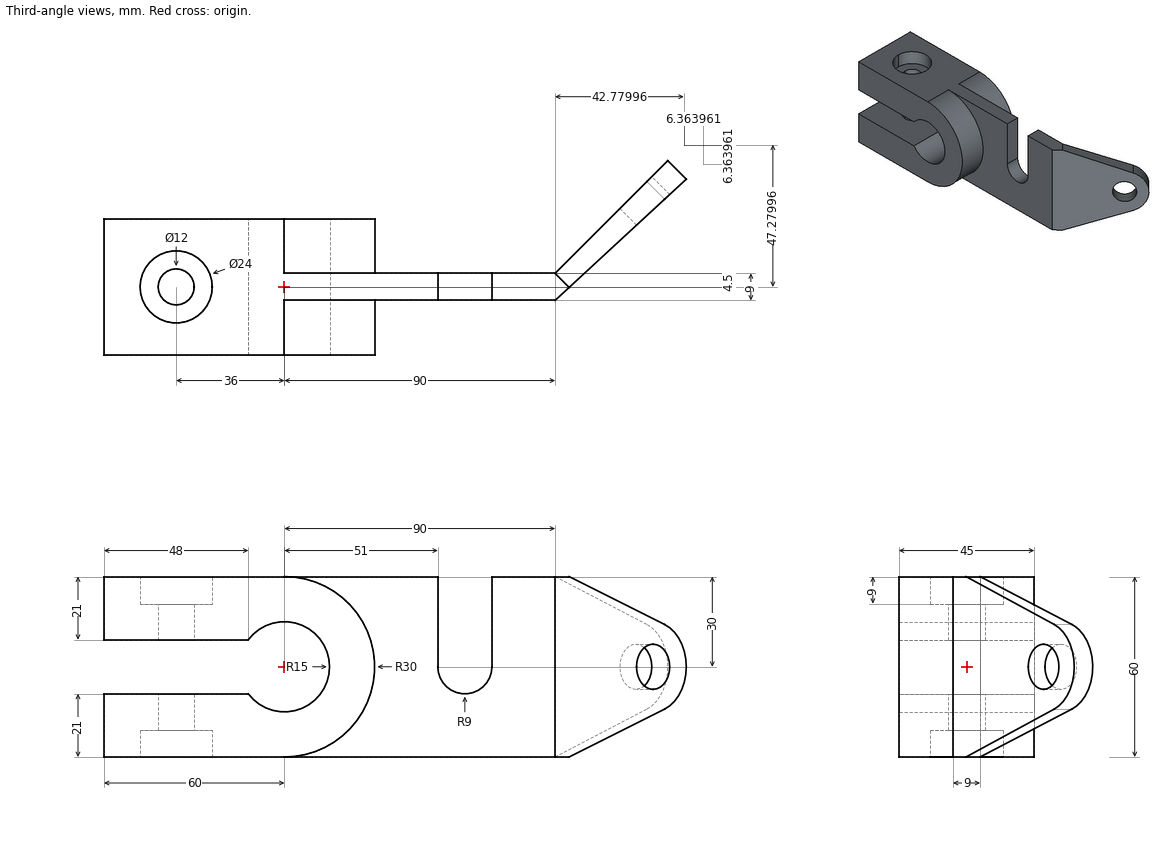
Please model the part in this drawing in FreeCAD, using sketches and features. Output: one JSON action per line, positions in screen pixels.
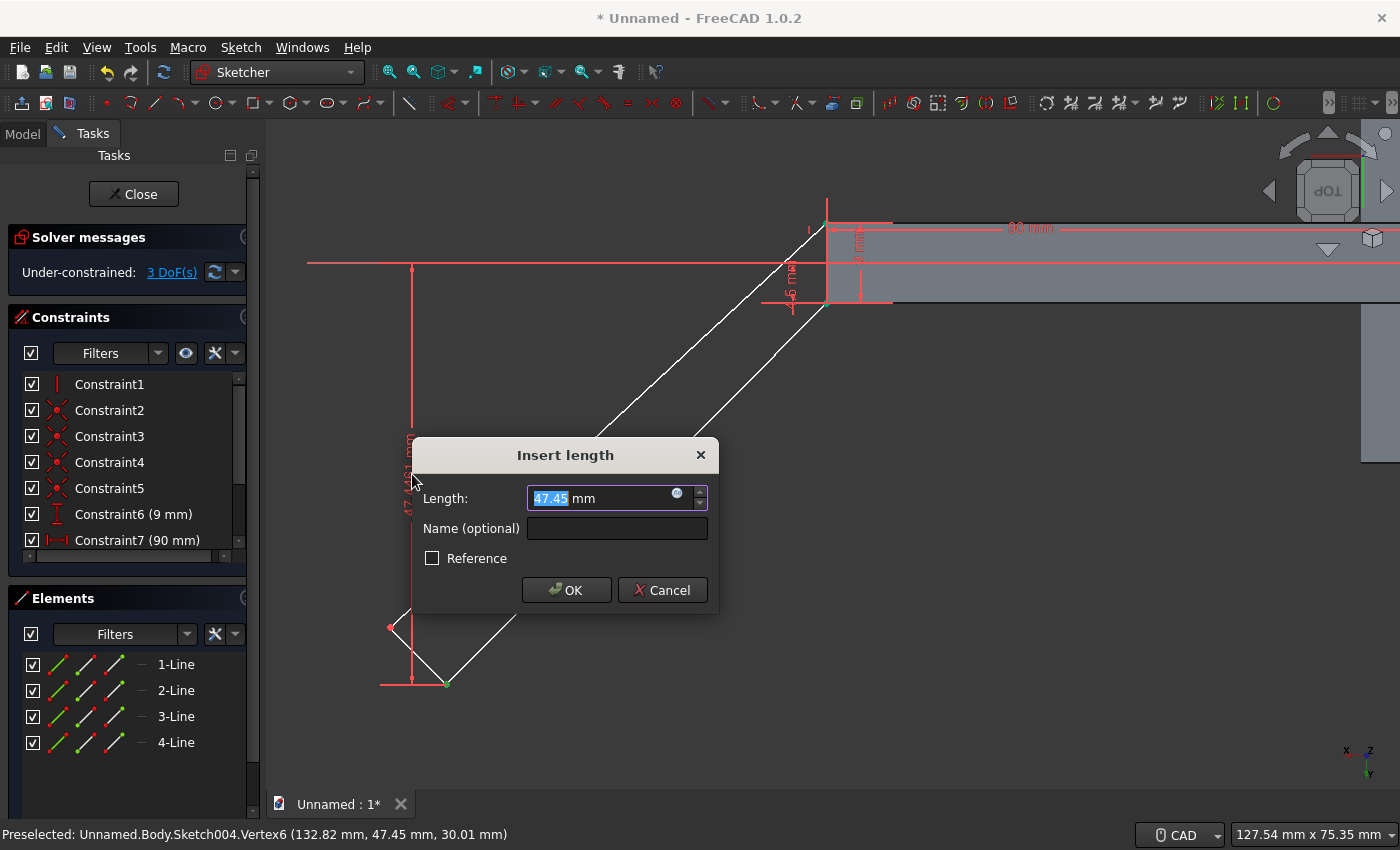
{"action": "type", "text": "47.27996"}
{"action": "key", "text": "Return"}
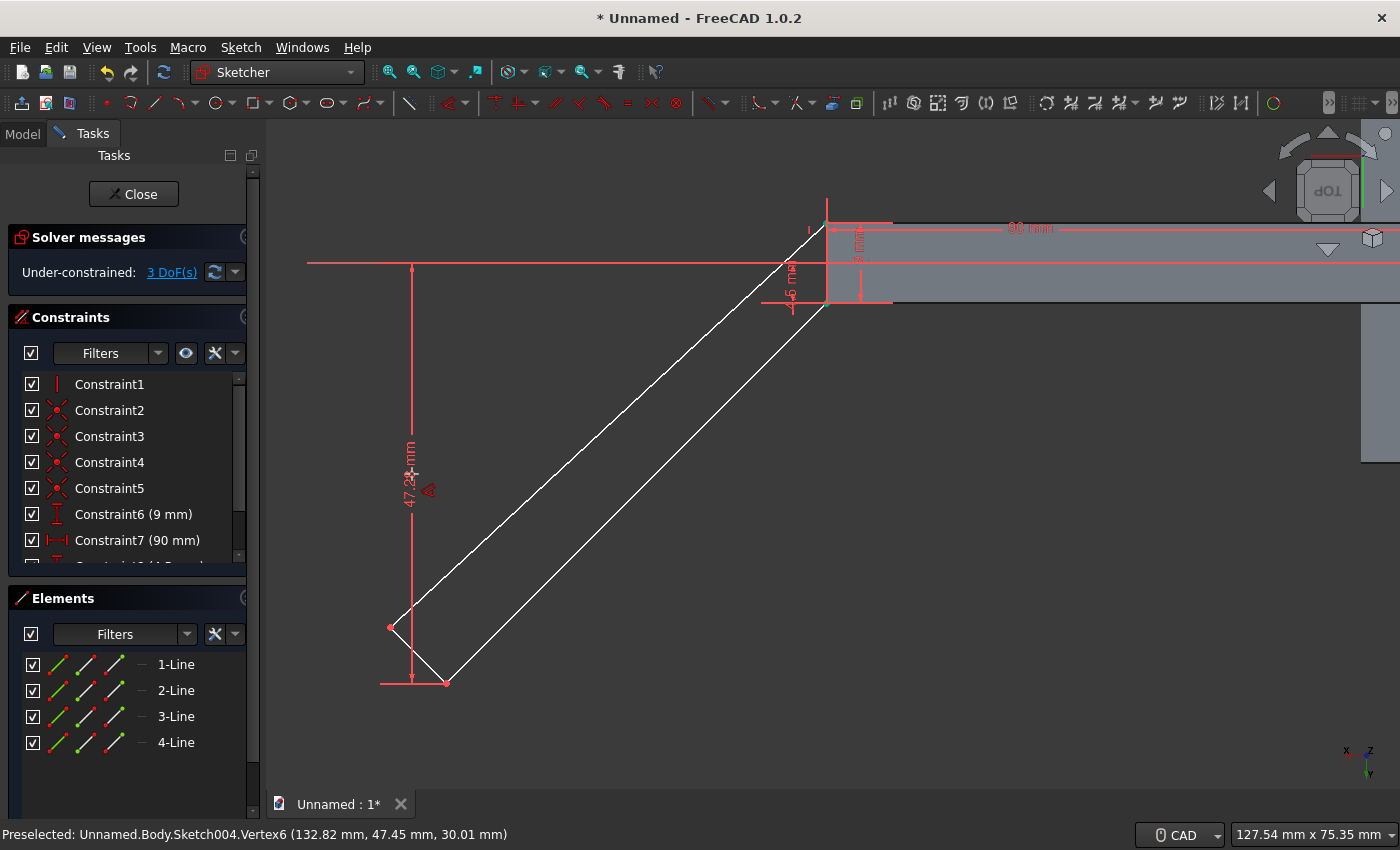
{"action": "left_click", "coordinate": [407, 645]}
{"action": "left_click", "coordinate": [418, 718]}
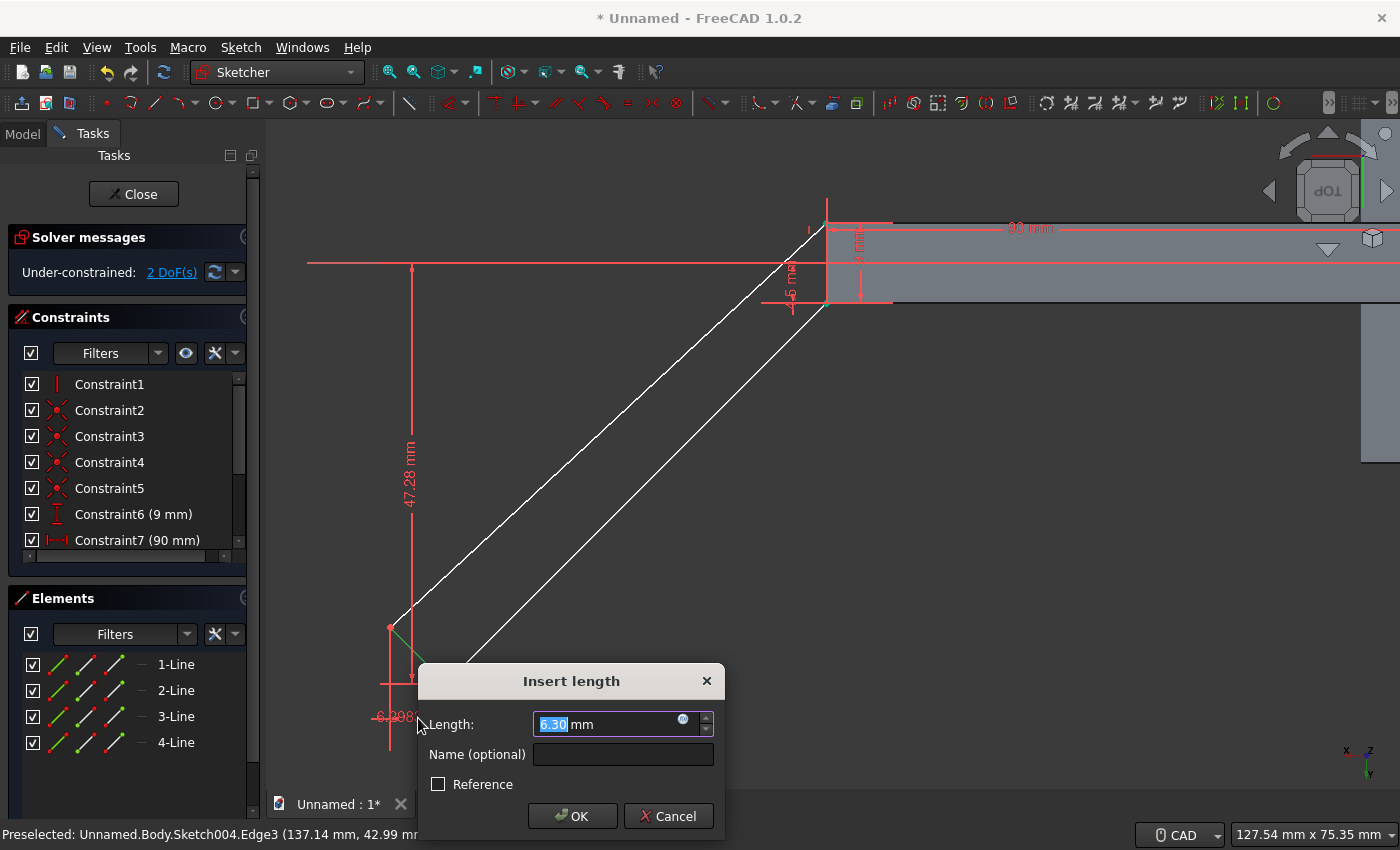
{"action": "type", "text": "6.363961"}
{"action": "key", "text": "Return"}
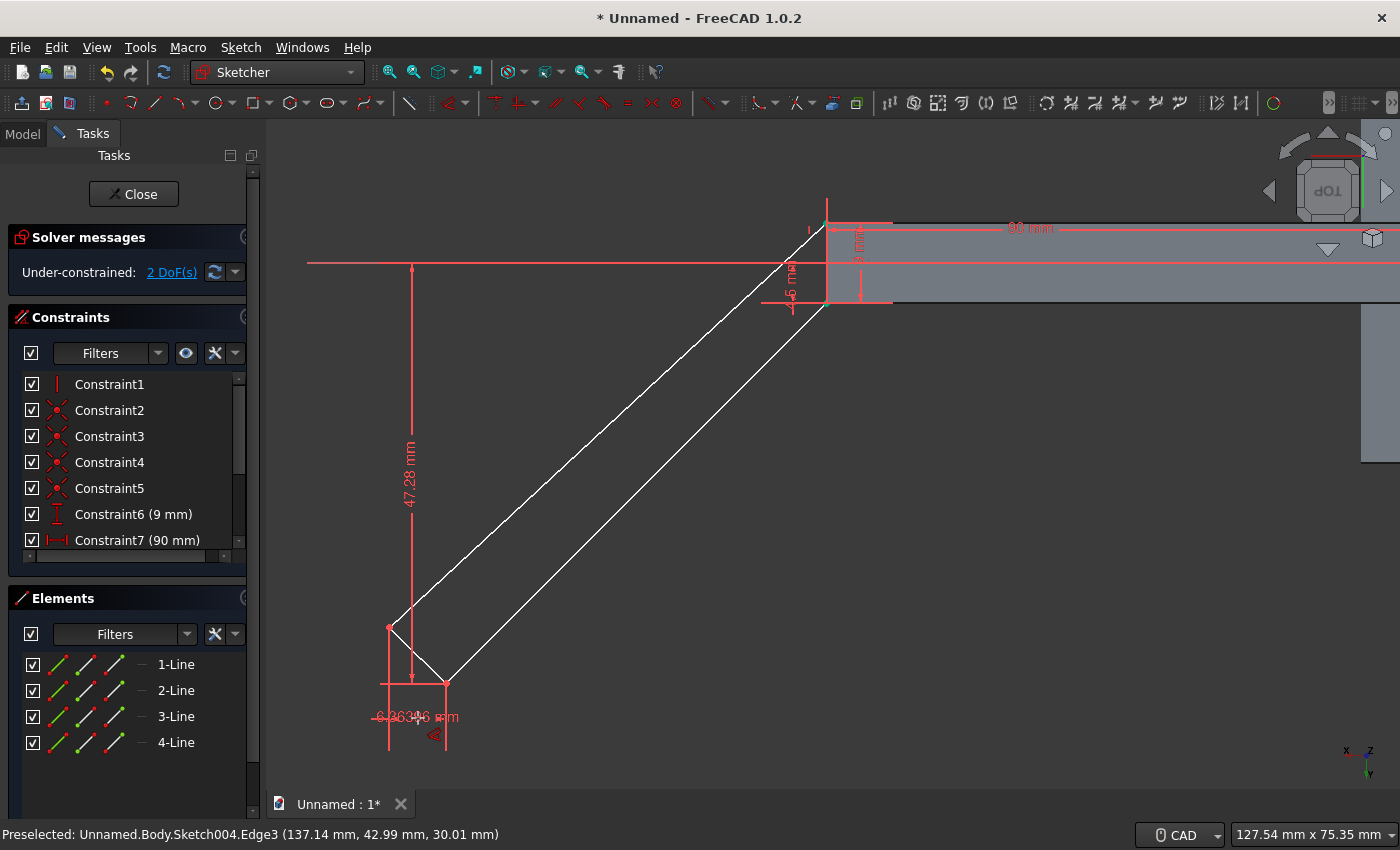
{"action": "left_click", "coordinate": [406, 645]}
{"action": "left_click", "coordinate": [355, 656]}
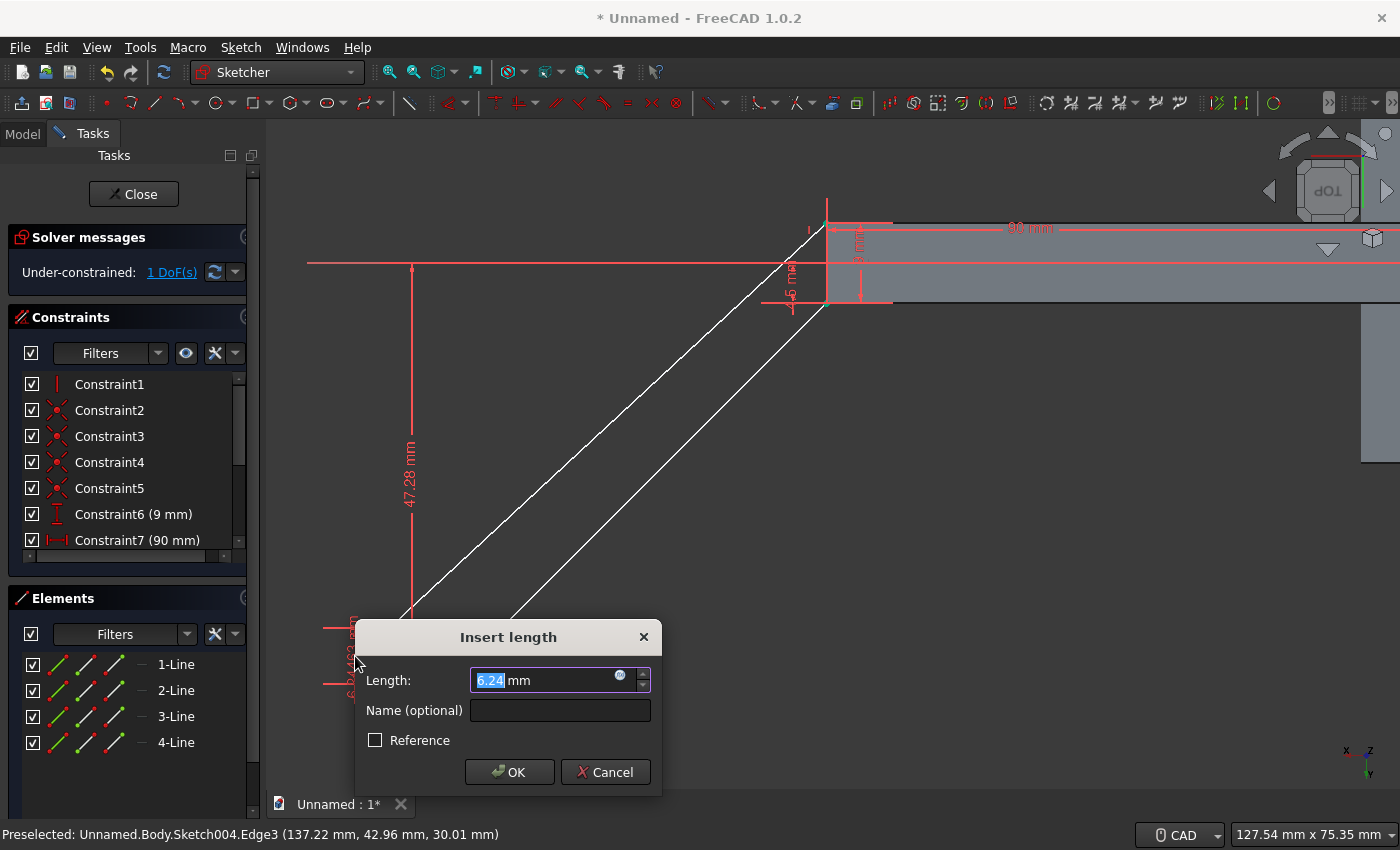
{"action": "type", "text": "6.363961"}
{"action": "key", "text": "Return"}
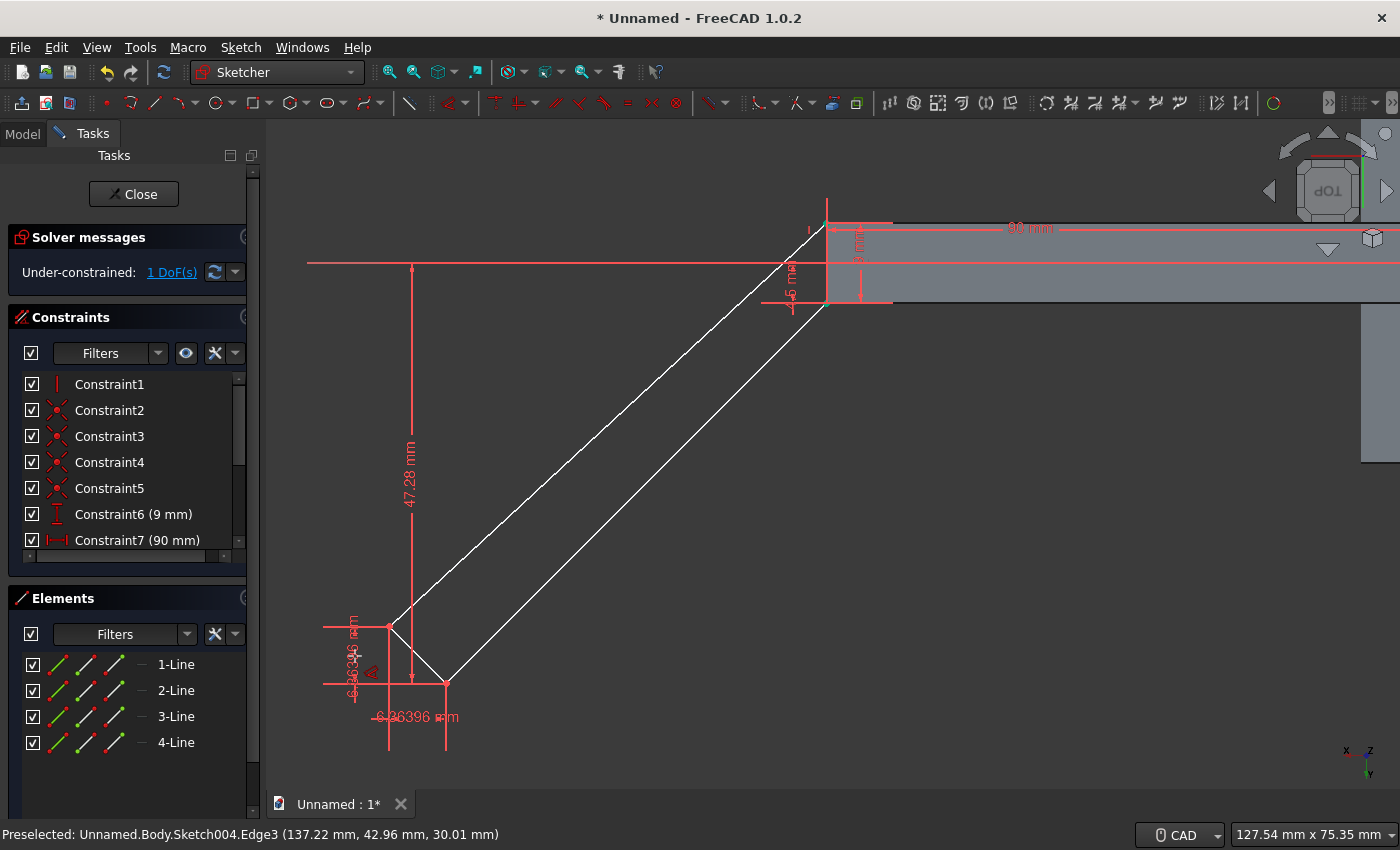
{"action": "left_click", "coordinate": [560, 569]}
{"action": "left_click", "coordinate": [636, 718]}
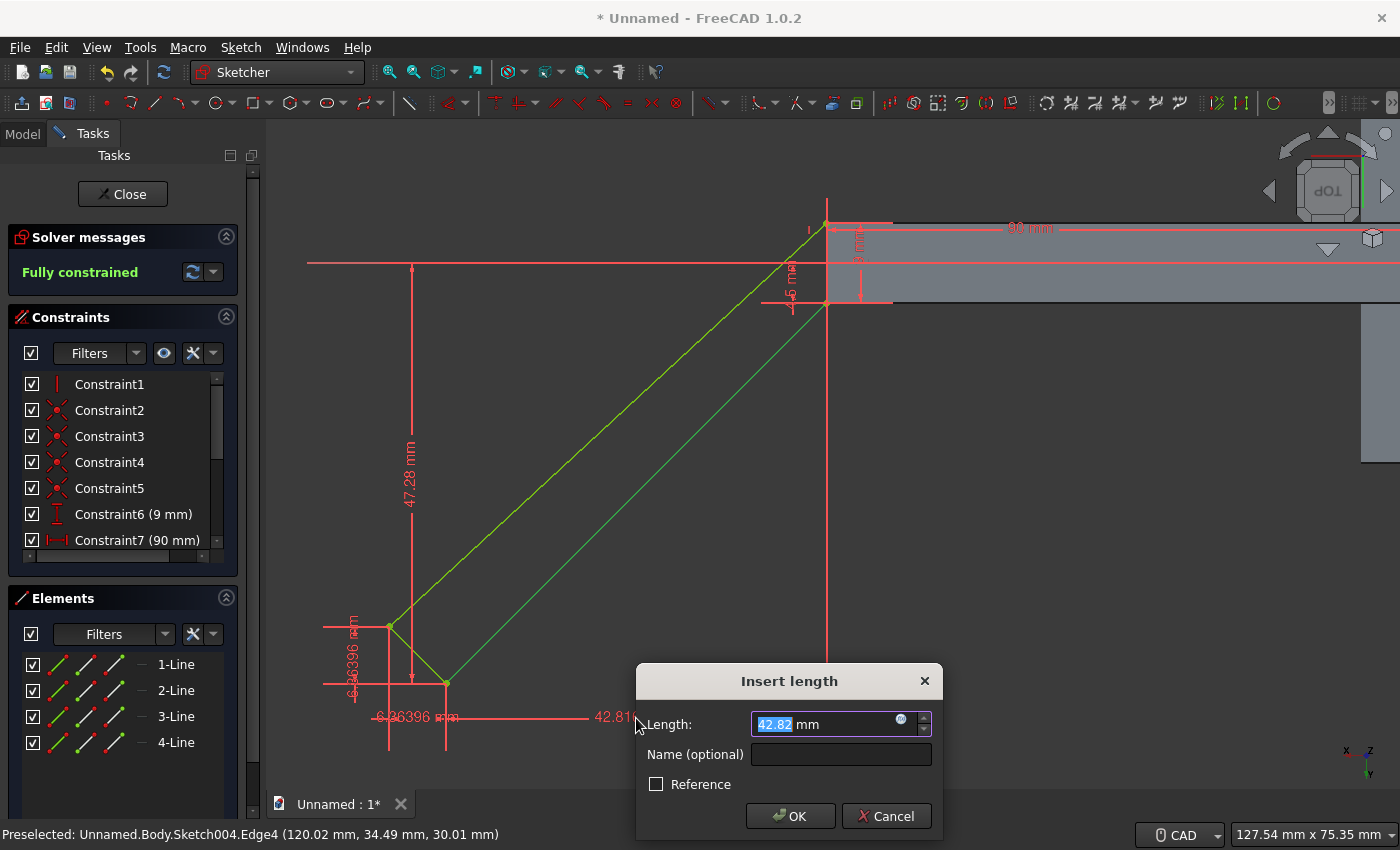
{"action": "type", "text": "42.77996"}
{"action": "key", "text": "Return"}
{"action": "key", "text": "Escape"}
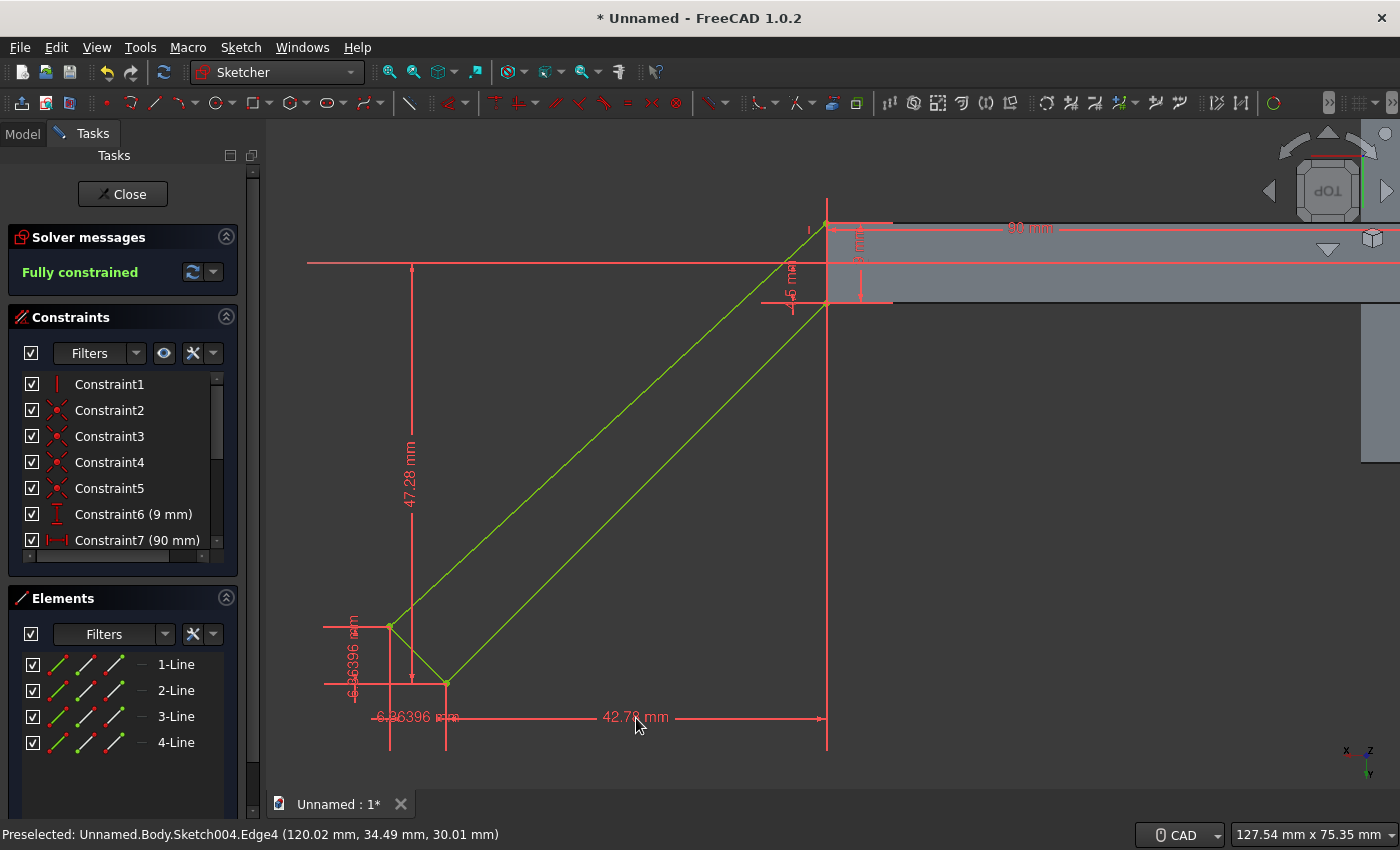
{"action": "left_click", "coordinate": [123, 194]}